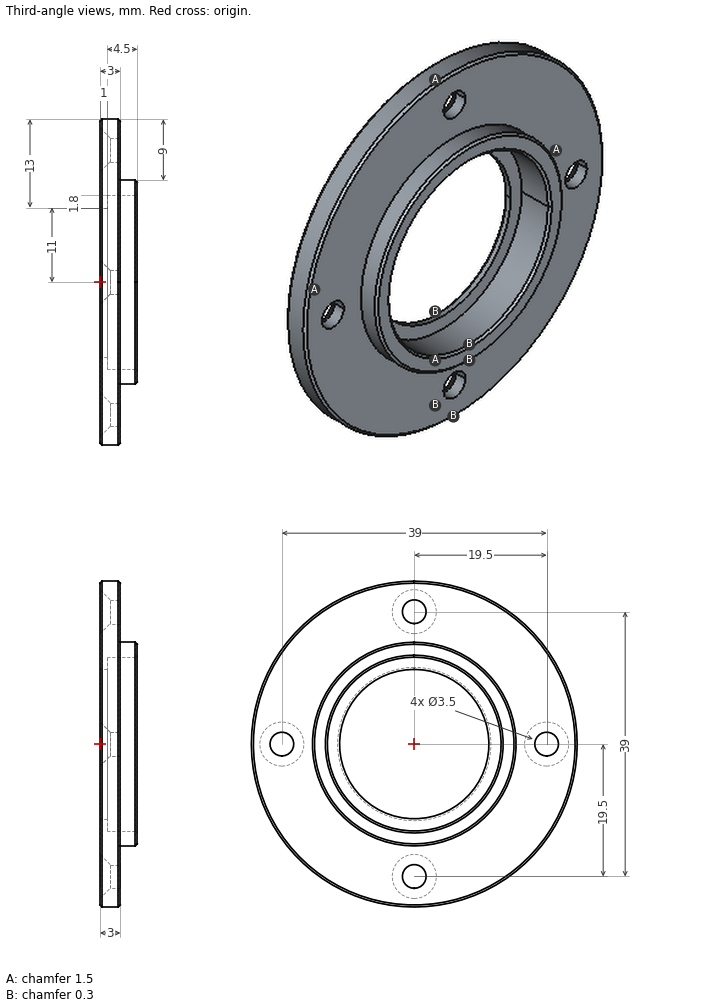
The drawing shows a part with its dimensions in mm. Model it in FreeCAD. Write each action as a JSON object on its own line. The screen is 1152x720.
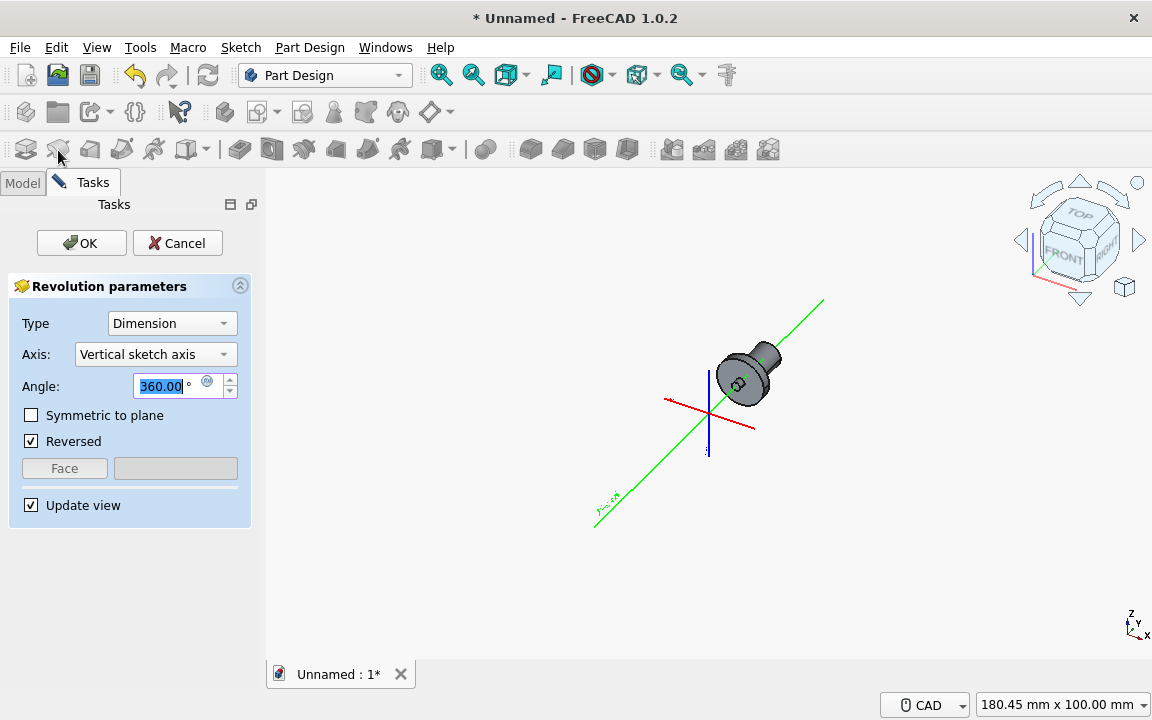
{"action": "left_click", "coordinate": [156, 354]}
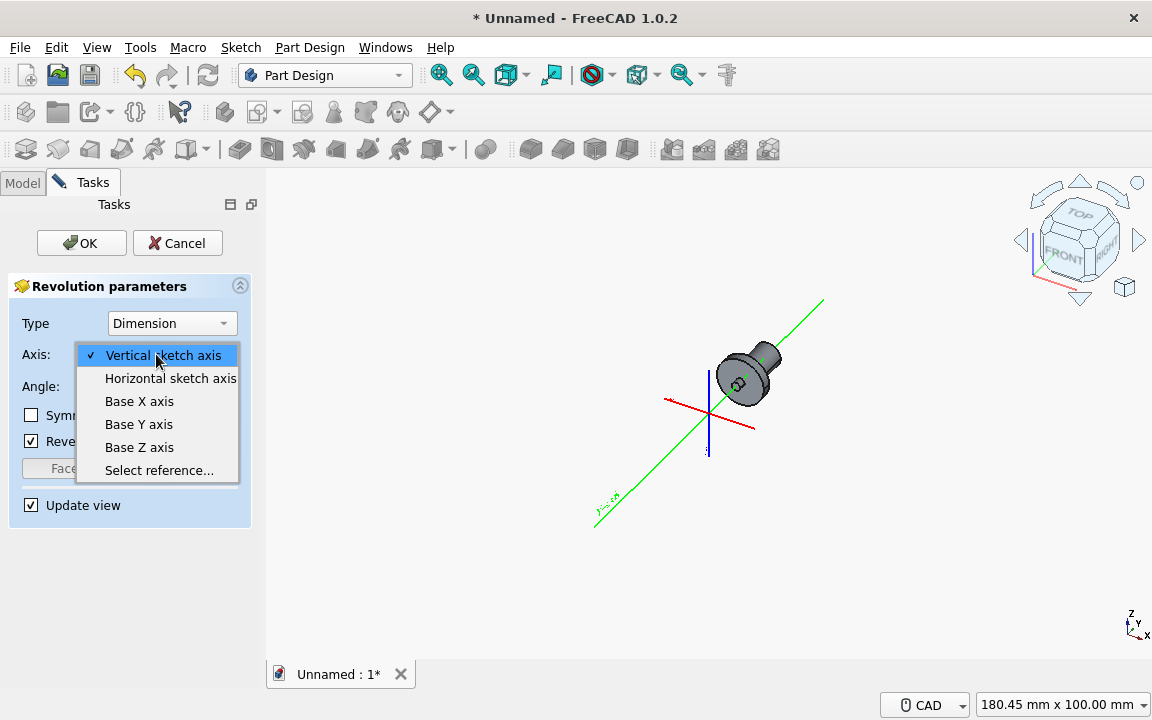
{"action": "left_click", "coordinate": [156, 378]}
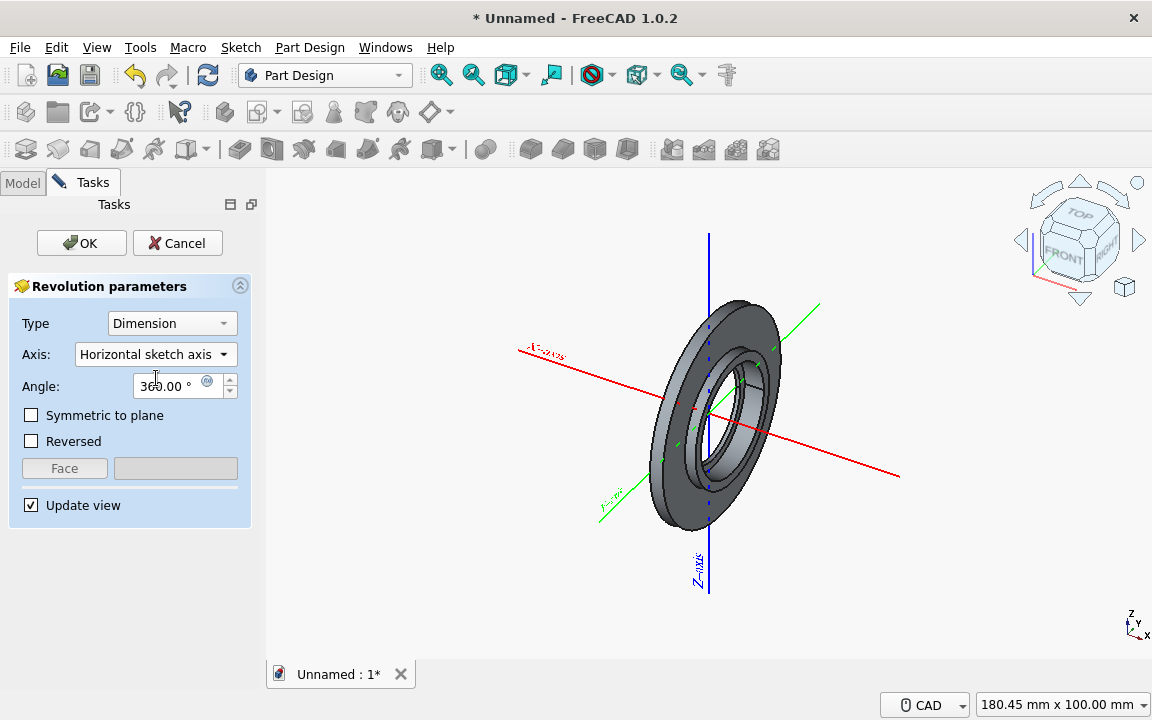
{"action": "left_click", "coordinate": [82, 243]}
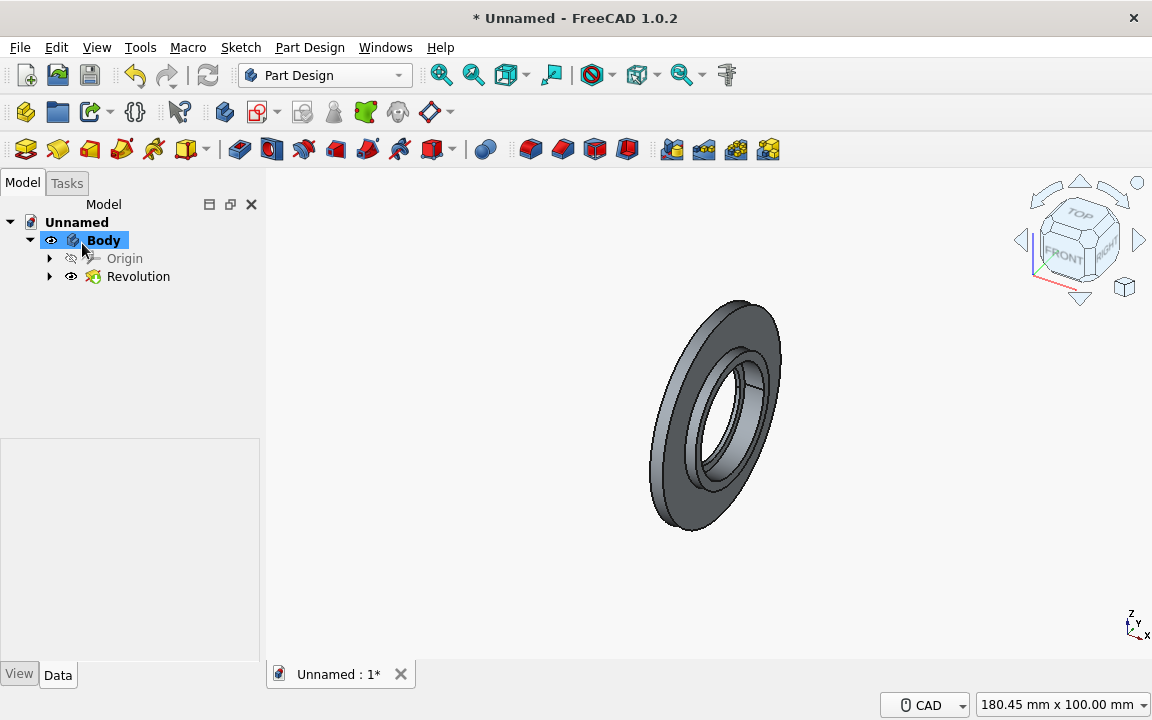
{"action": "left_click", "coordinate": [688, 395]}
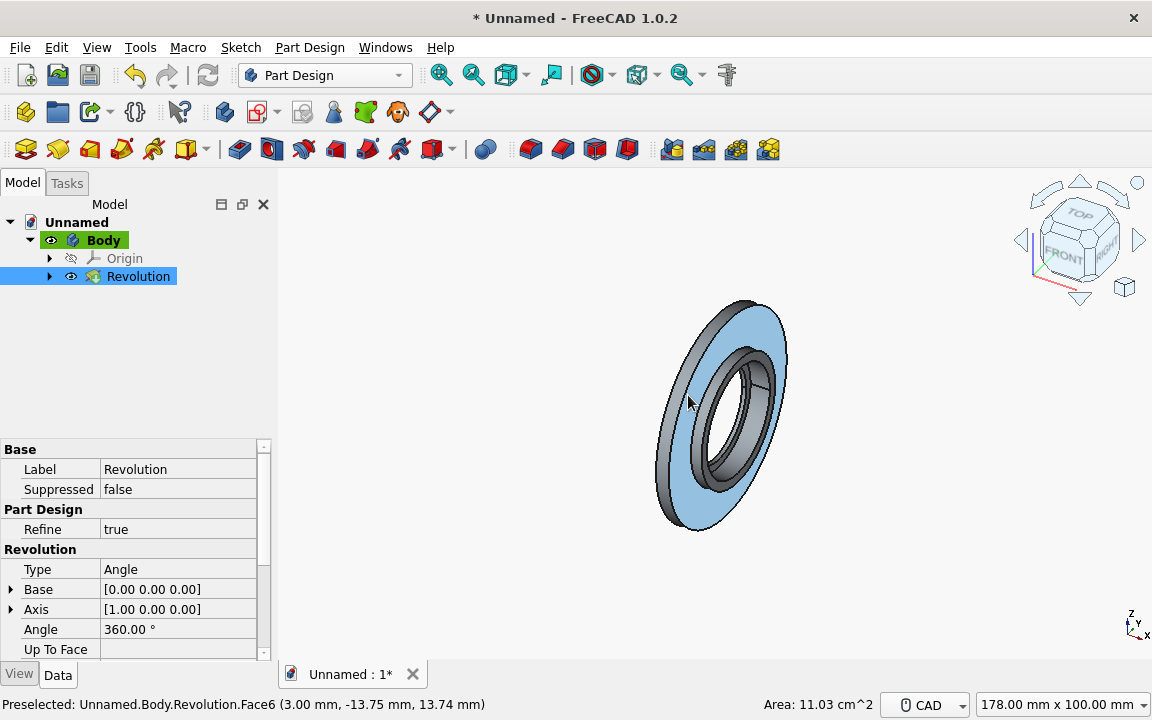
{"action": "left_click", "coordinate": [258, 112]}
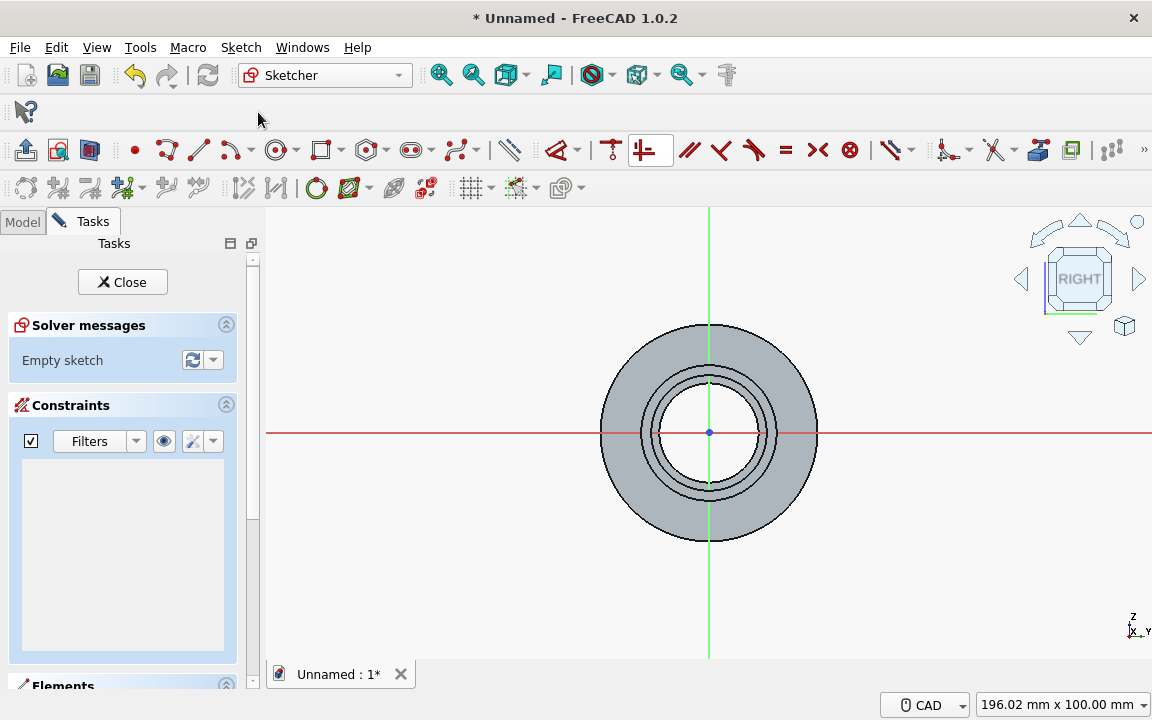
{"action": "scroll", "coordinate": [848, 433], "scroll_direction": "up", "scroll_amount": 2}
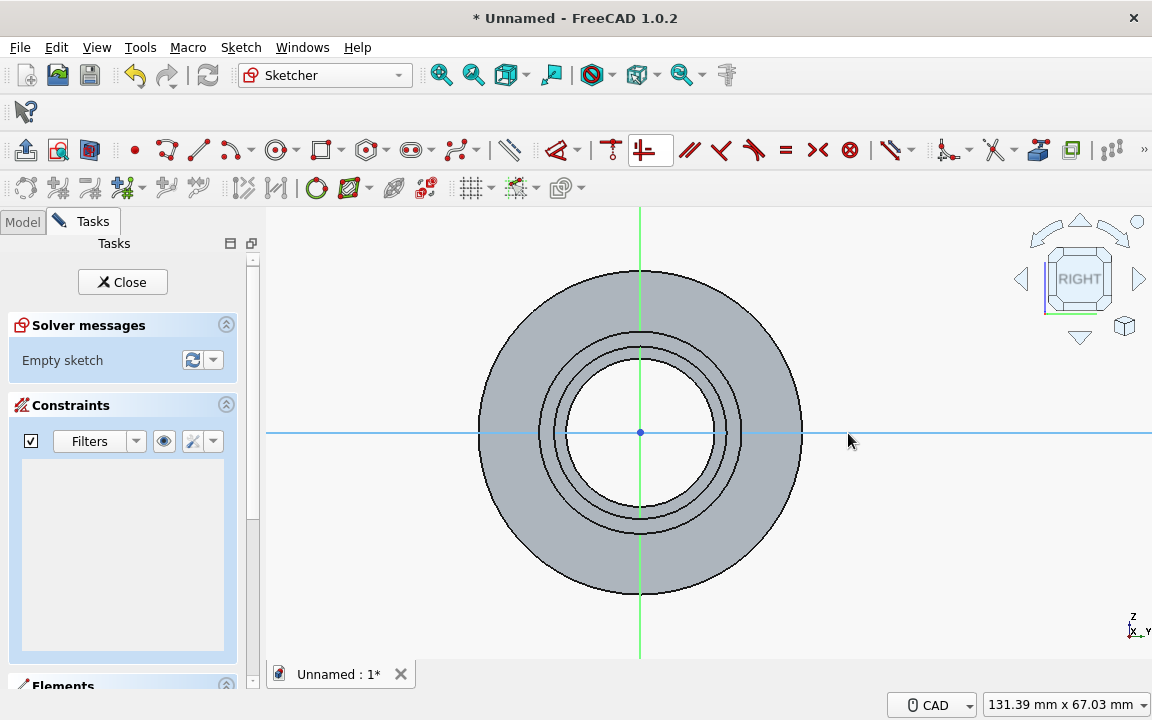
{"action": "left_click", "coordinate": [276, 150]}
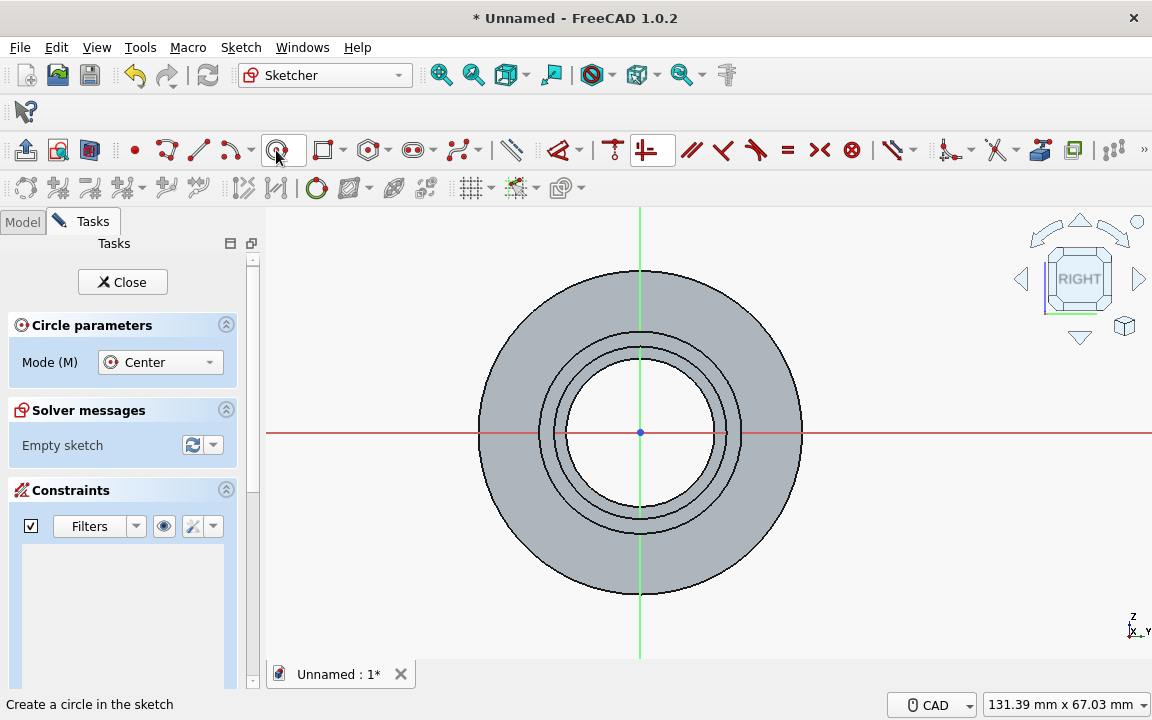
{"action": "scroll", "coordinate": [772, 433], "scroll_direction": "up", "scroll_amount": 4}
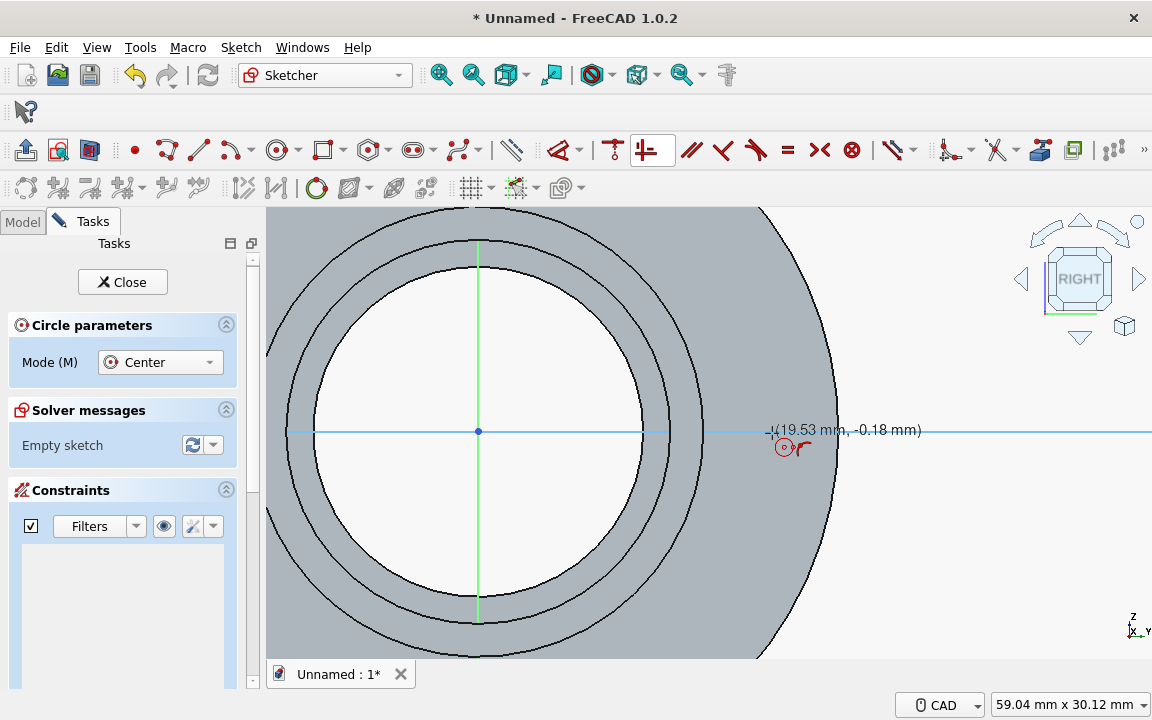
{"action": "left_click", "coordinate": [771, 432]}
{"action": "mouse_move", "coordinate": [789, 413]}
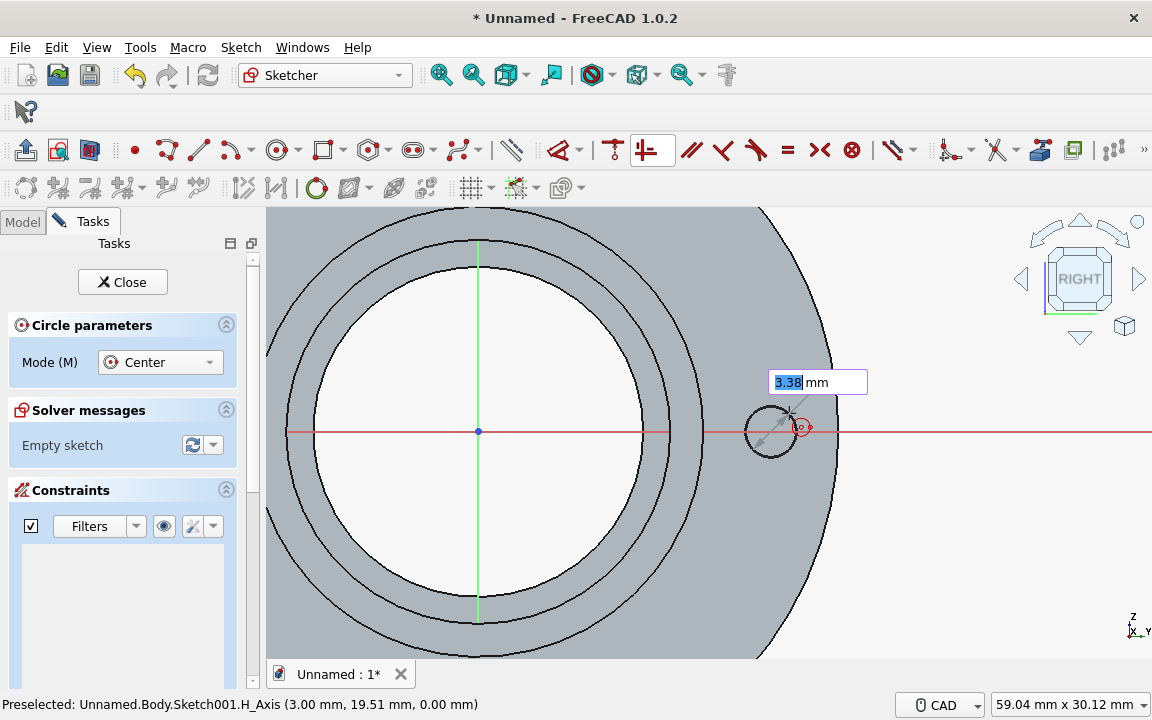
{"action": "type", "text": "3.5"}
{"action": "key", "text": "Return"}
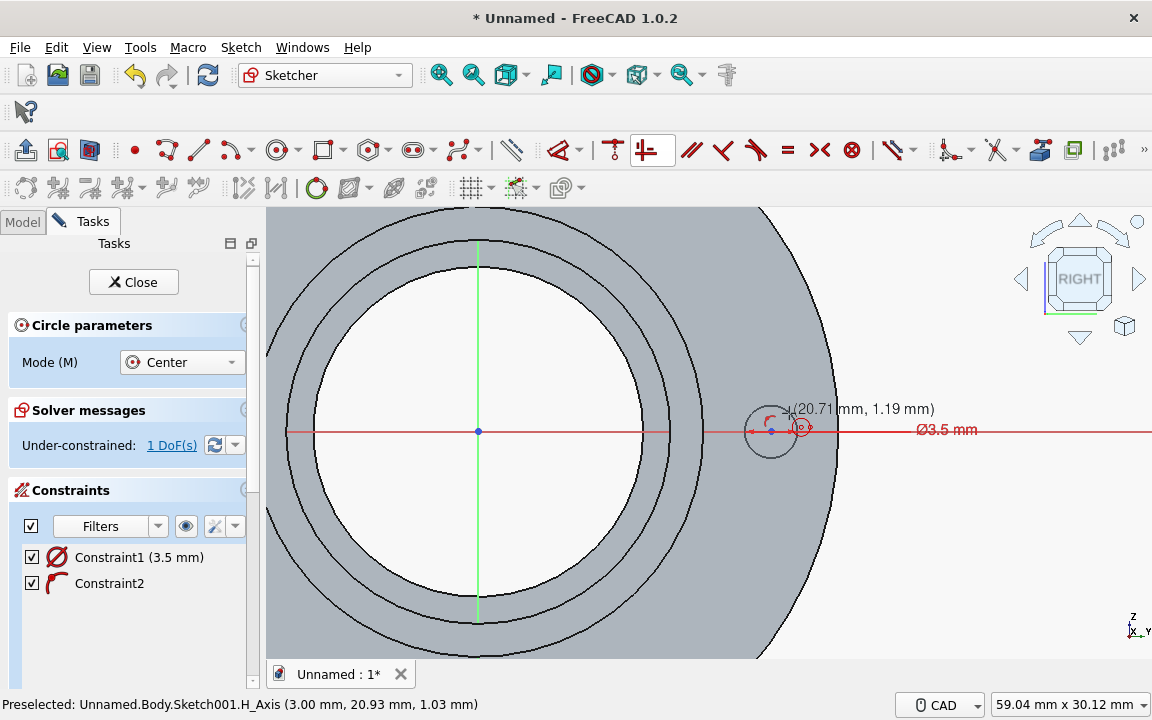
{"action": "scroll", "coordinate": [773, 434], "scroll_direction": "down", "scroll_amount": 4}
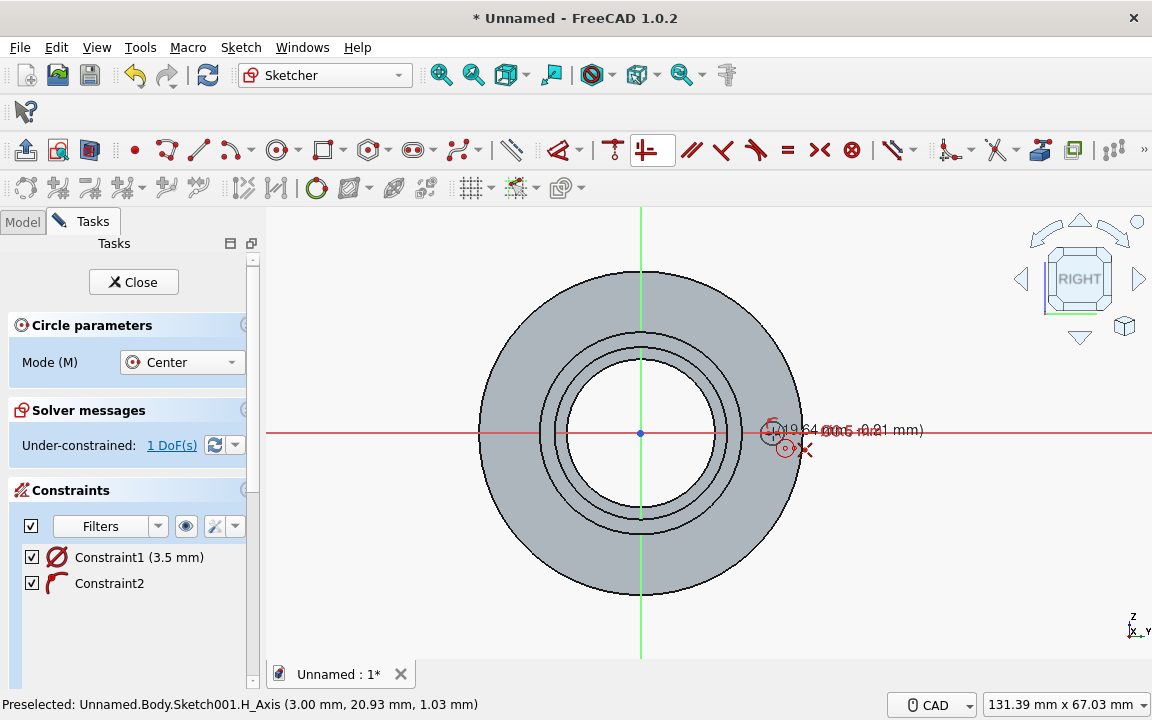
{"action": "scroll", "coordinate": [641, 565], "scroll_direction": "up", "scroll_amount": 4}